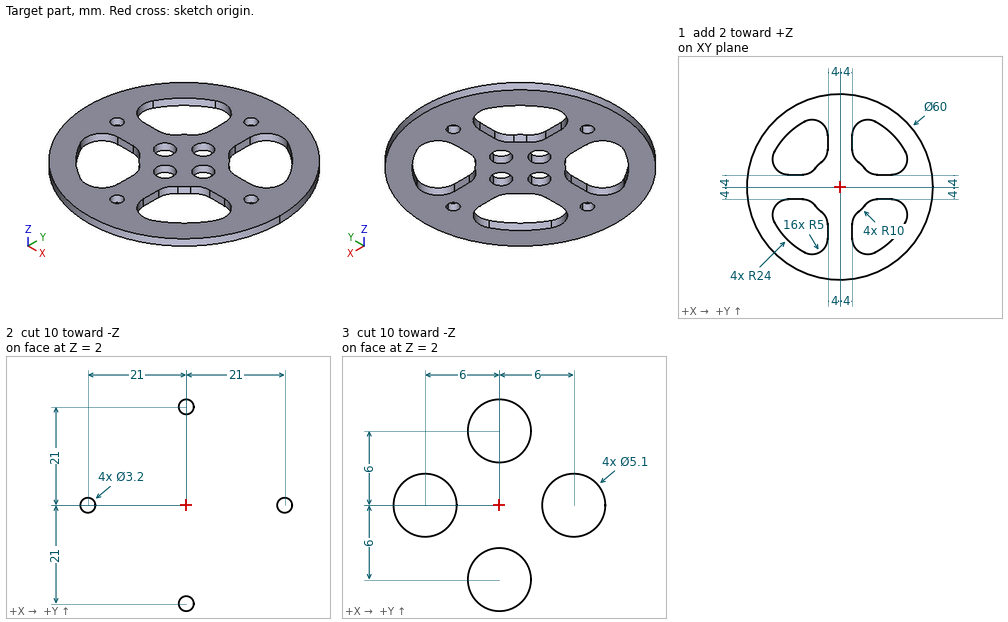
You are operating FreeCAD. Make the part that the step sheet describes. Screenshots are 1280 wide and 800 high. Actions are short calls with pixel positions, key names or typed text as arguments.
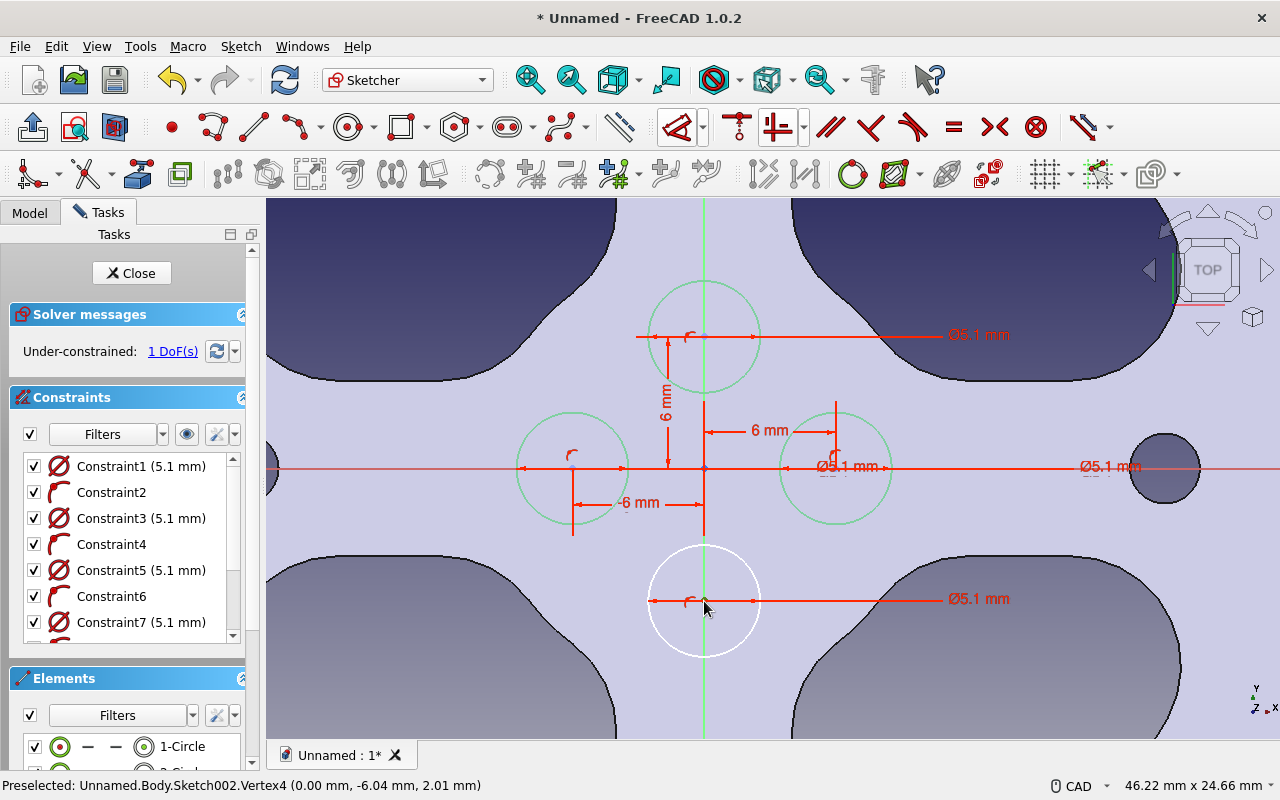
key(i)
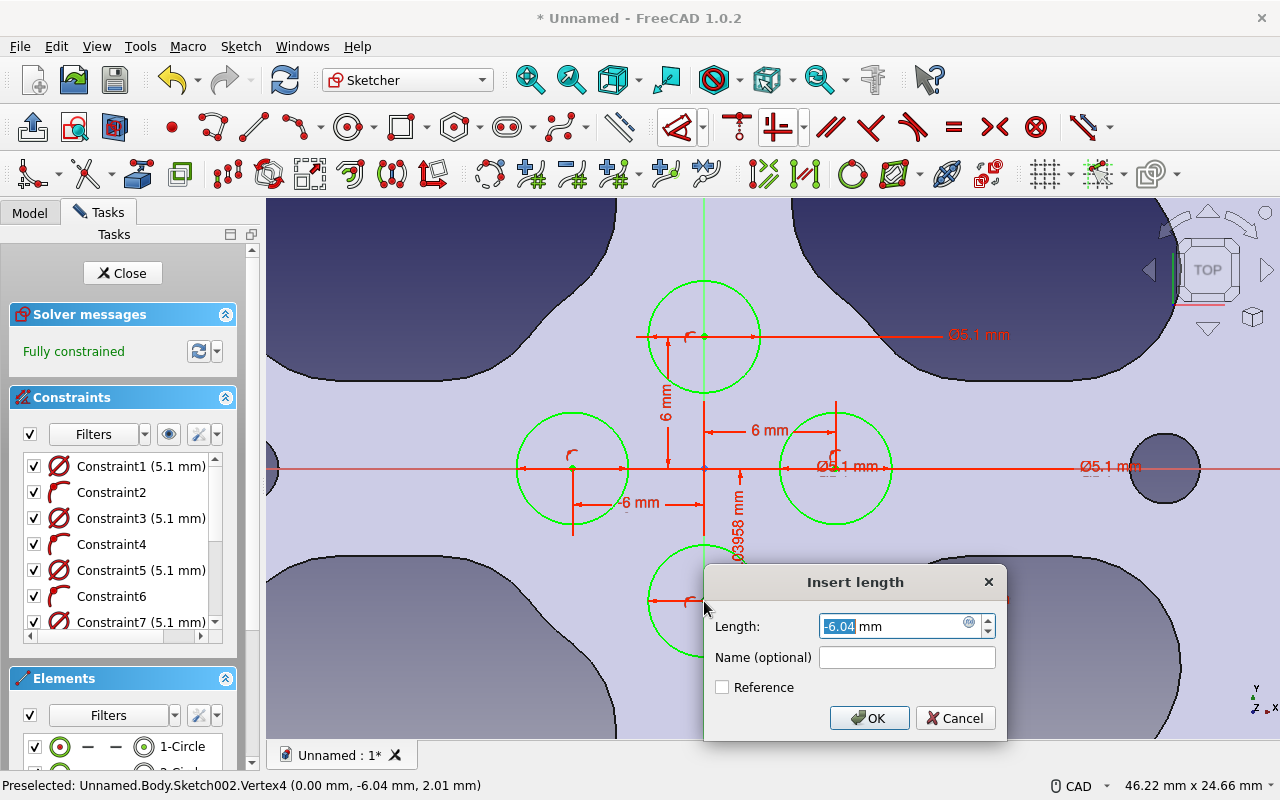
text(-6)
key(Return)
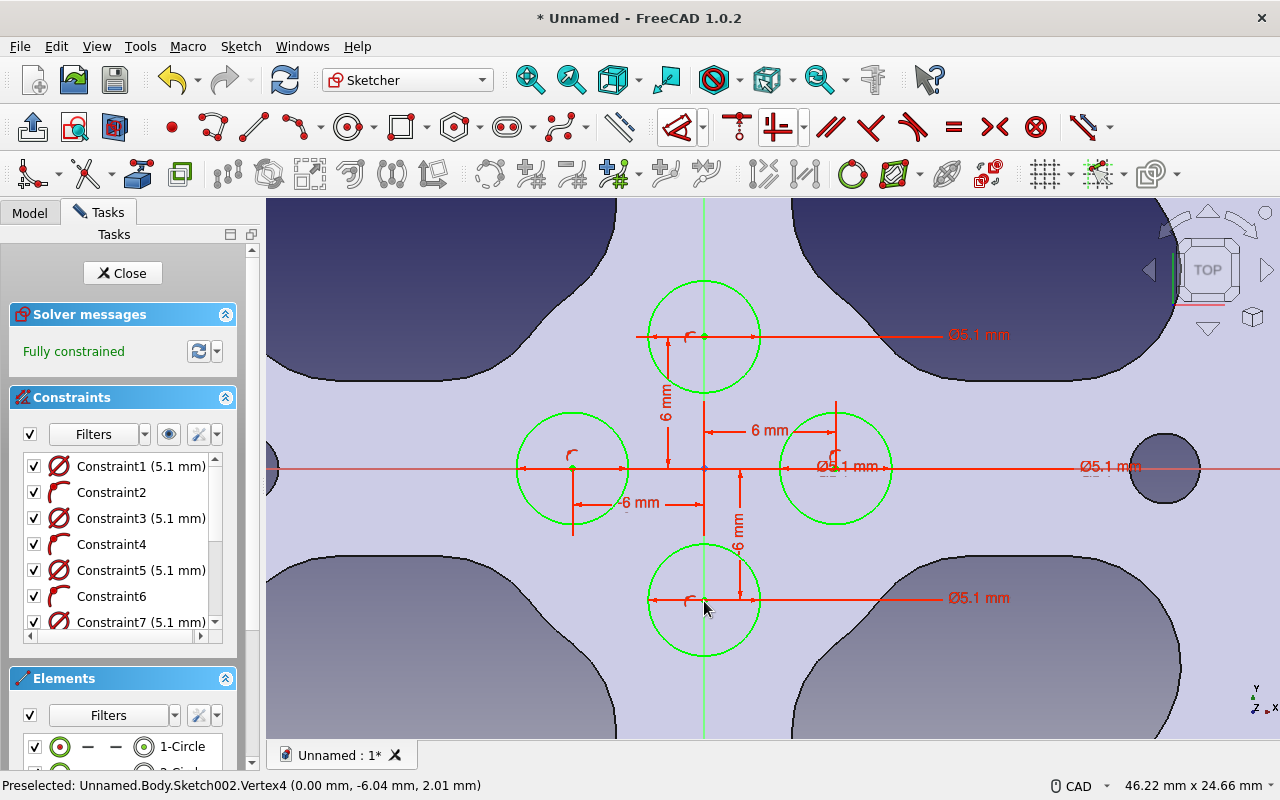
click(123, 273)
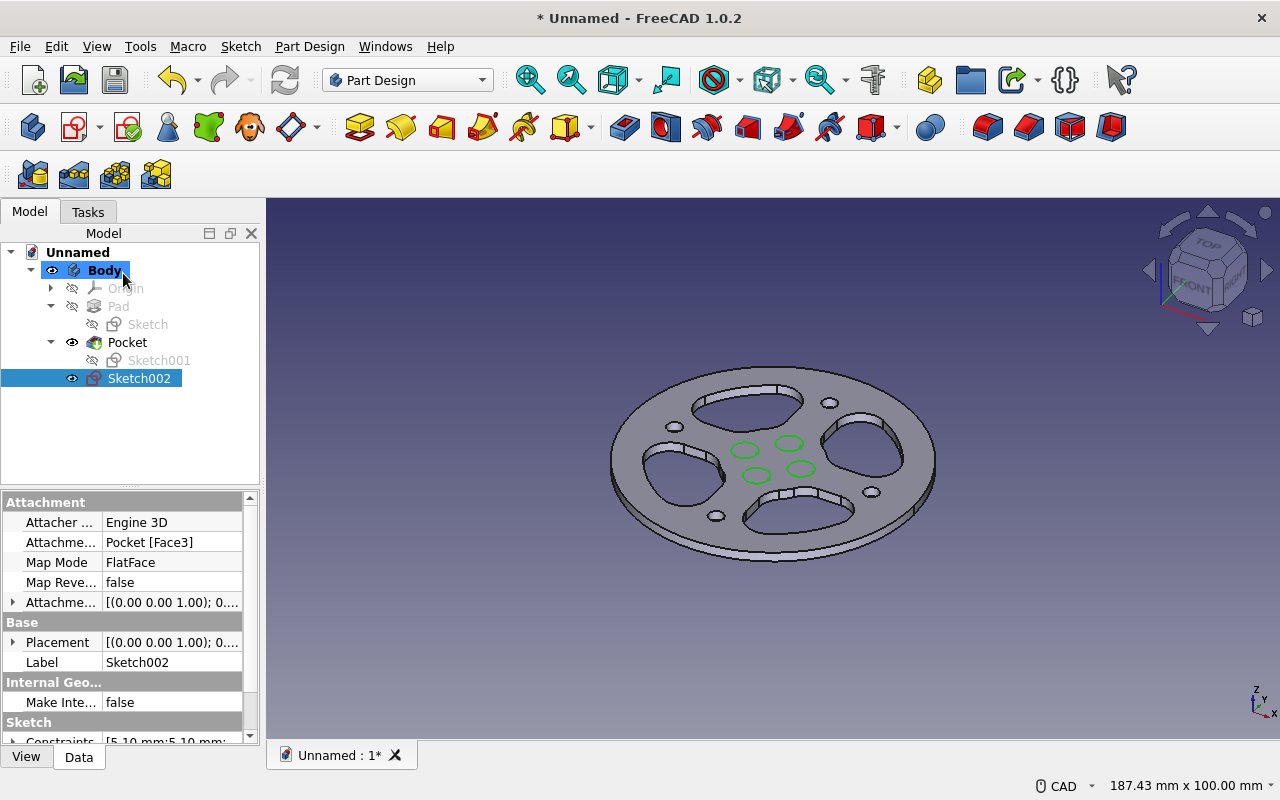
click(625, 128)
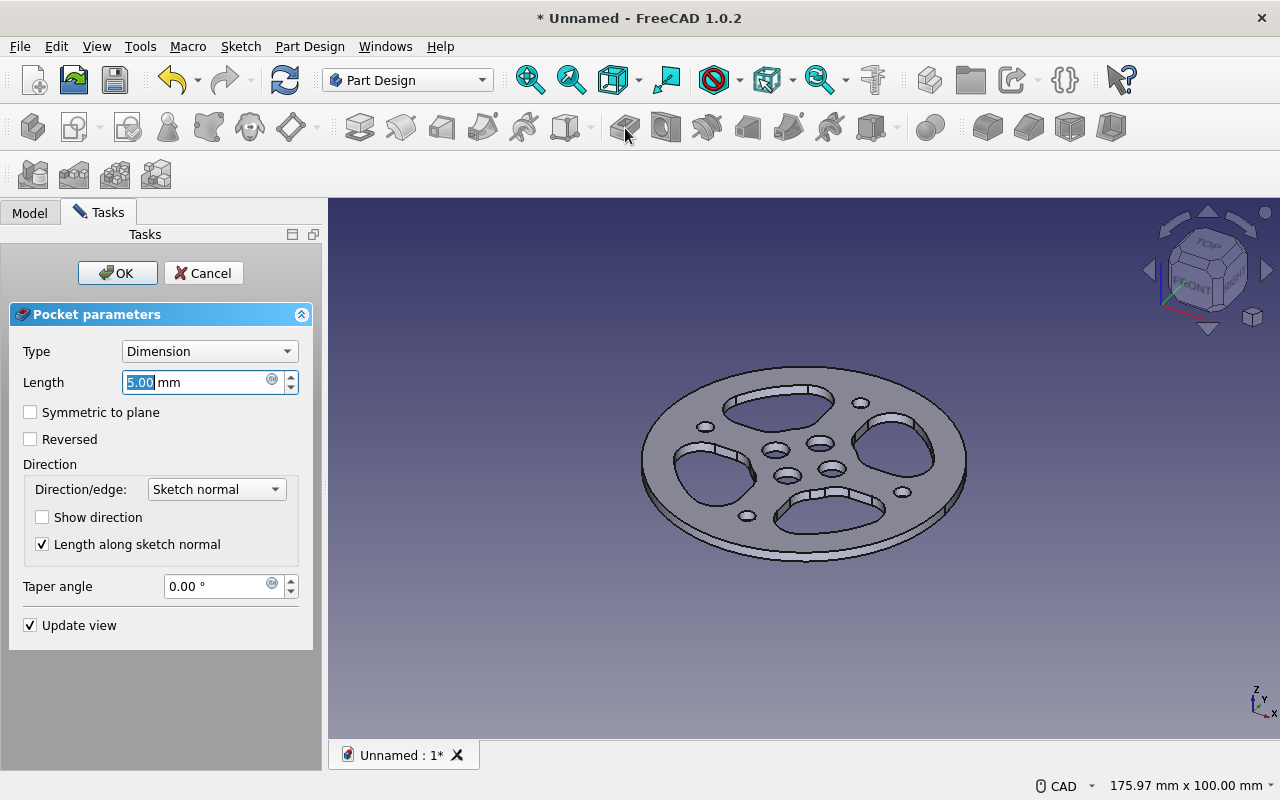
text(10)
key(Tab)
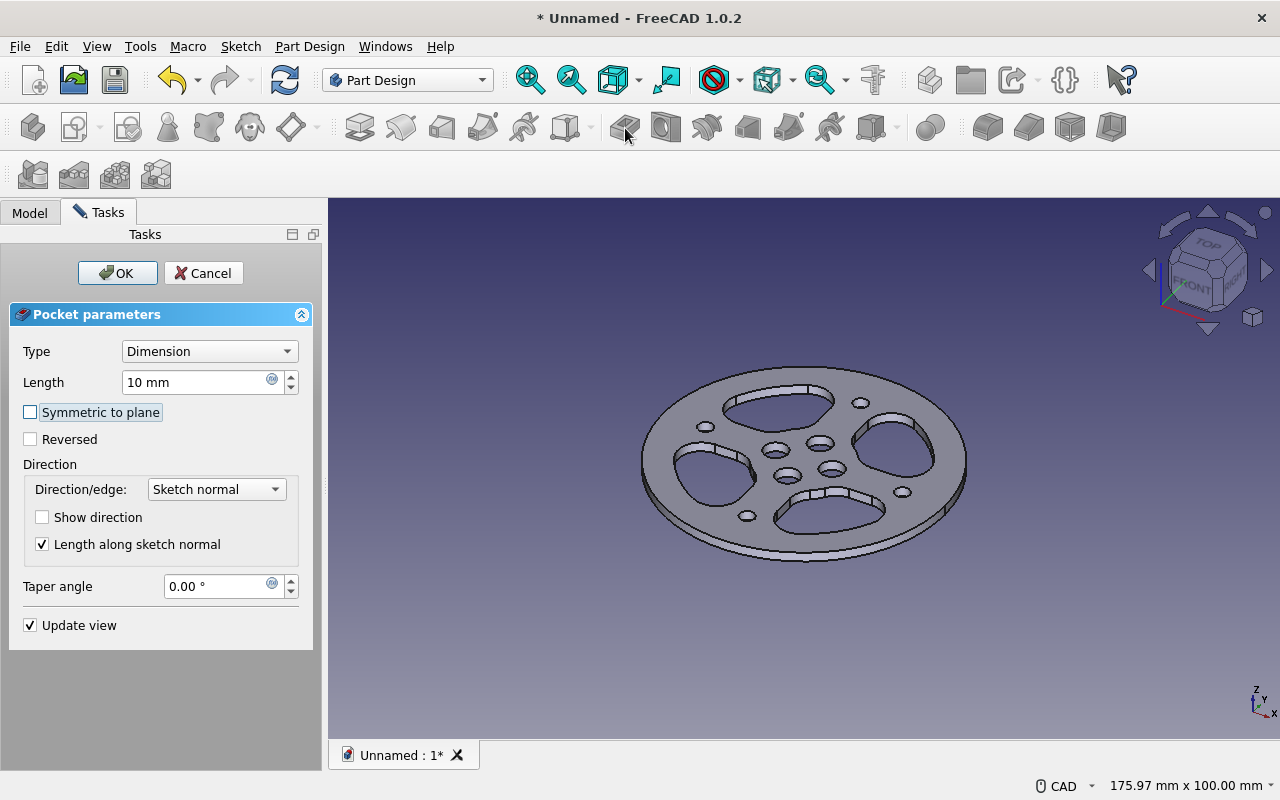
click(118, 273)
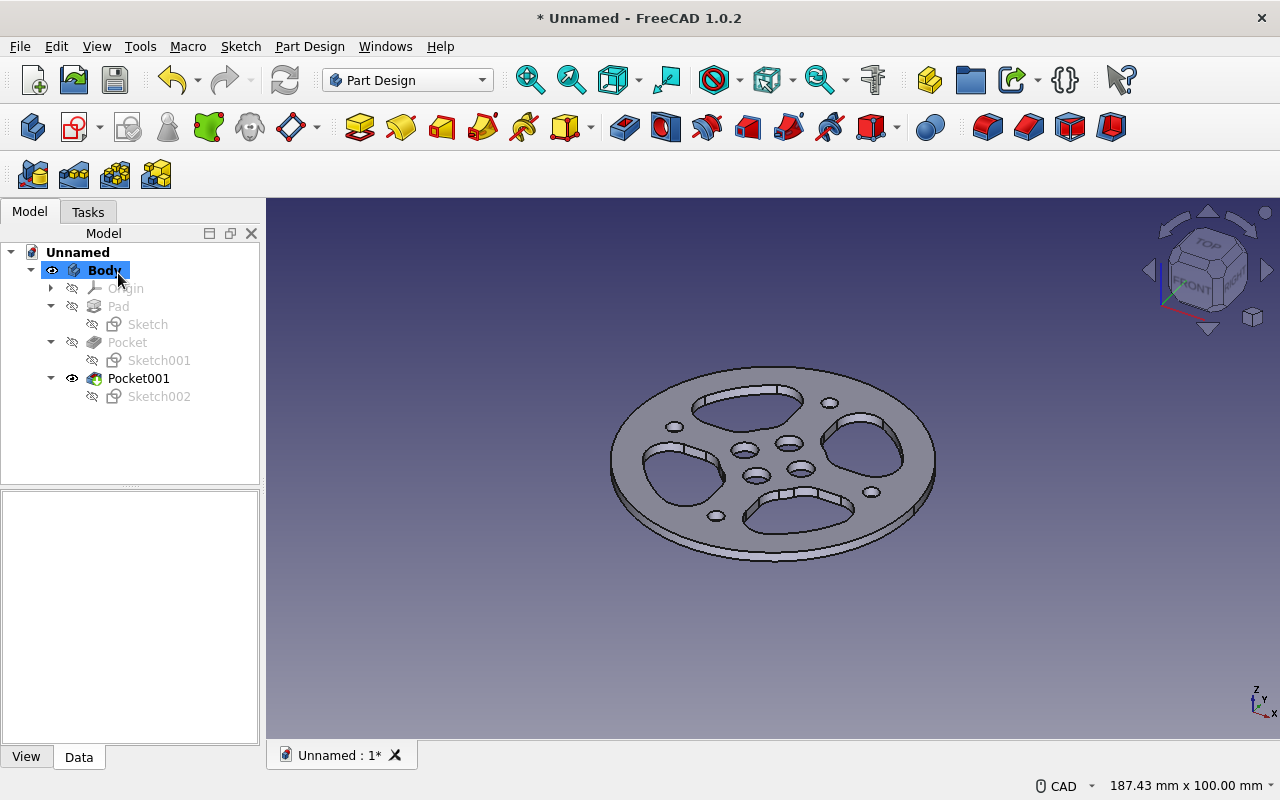
key(0)